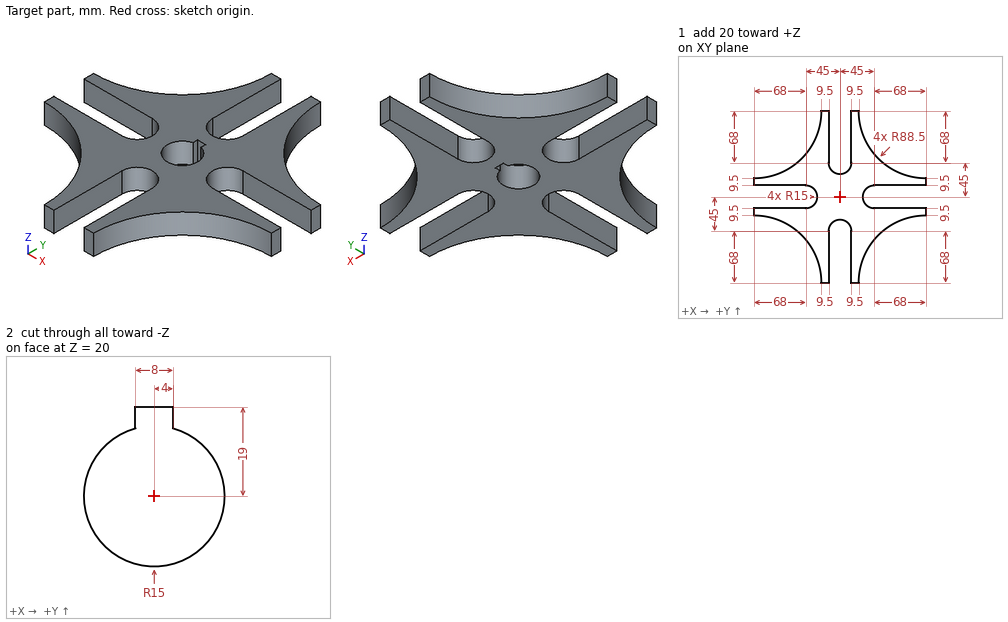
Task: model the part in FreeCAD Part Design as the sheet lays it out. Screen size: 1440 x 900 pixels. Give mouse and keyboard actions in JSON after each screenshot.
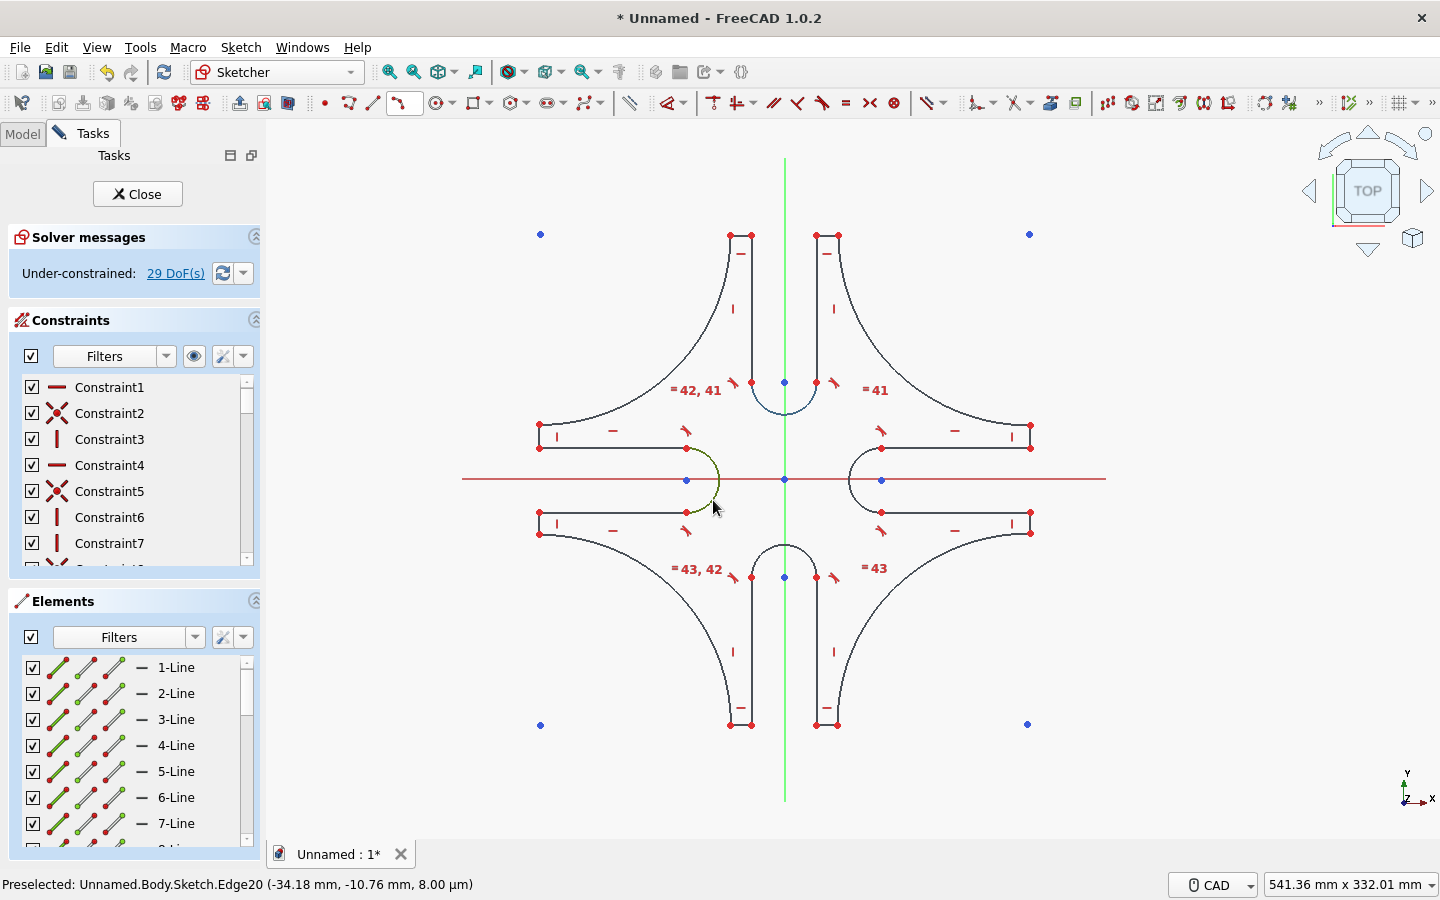
{"action": "left_click", "coordinate": [803, 551]}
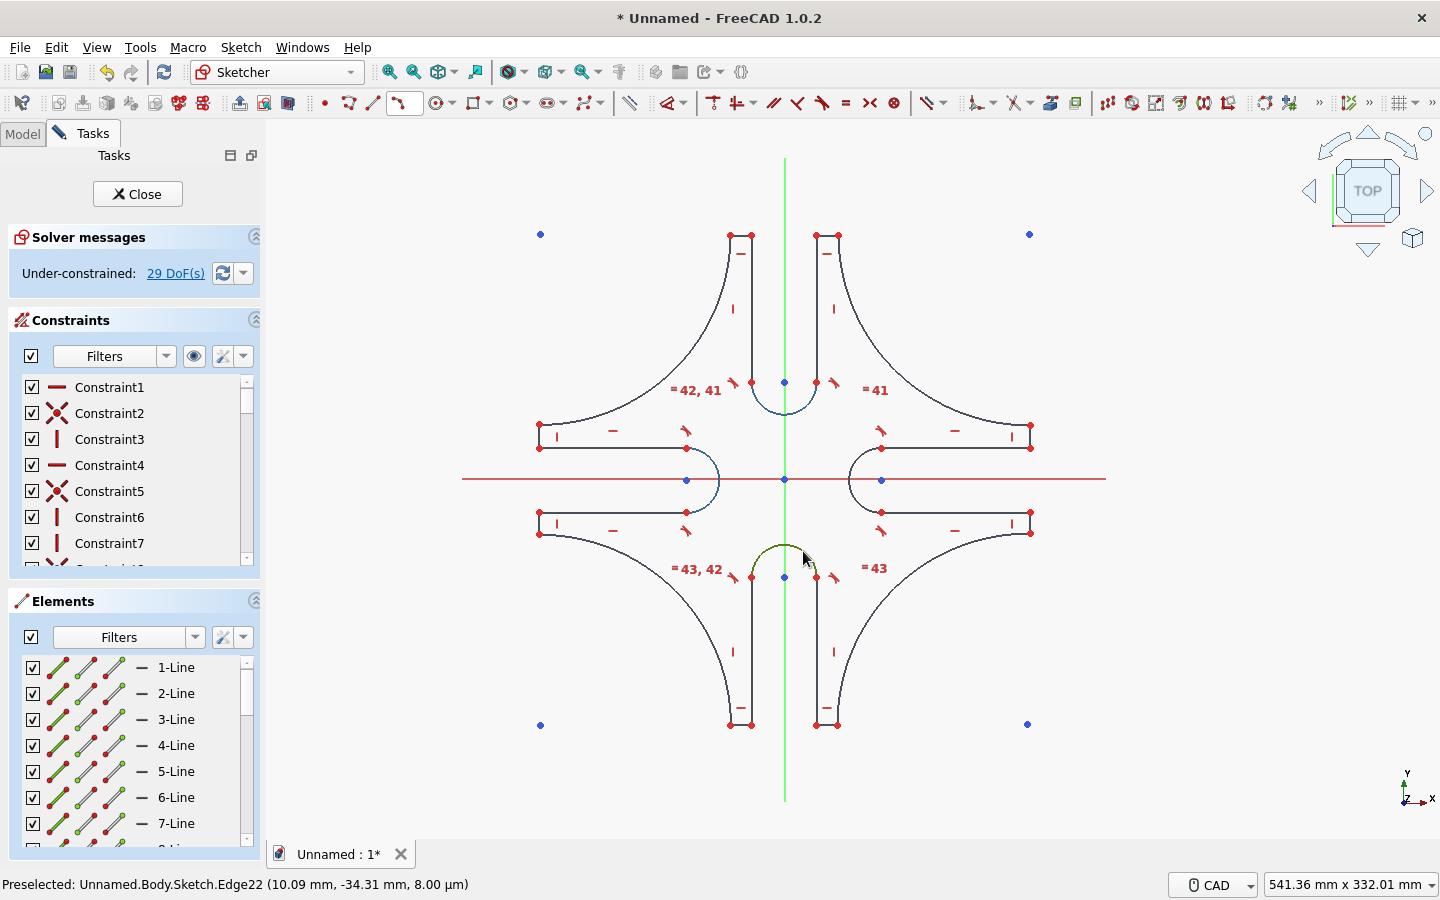
{"action": "left_click", "coordinate": [855, 461]}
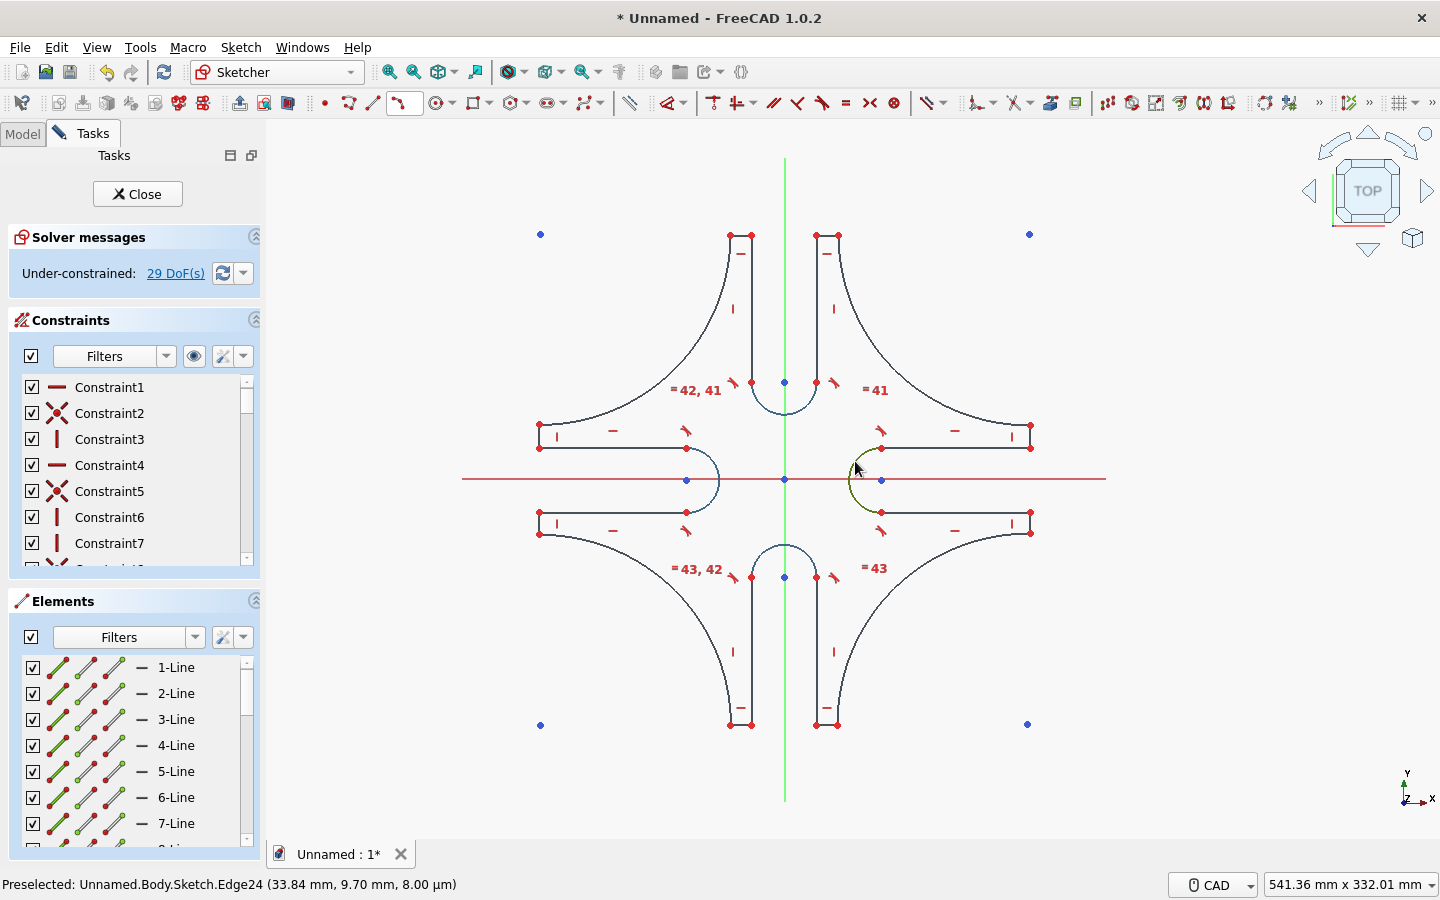
{"action": "left_click", "coordinate": [846, 104]}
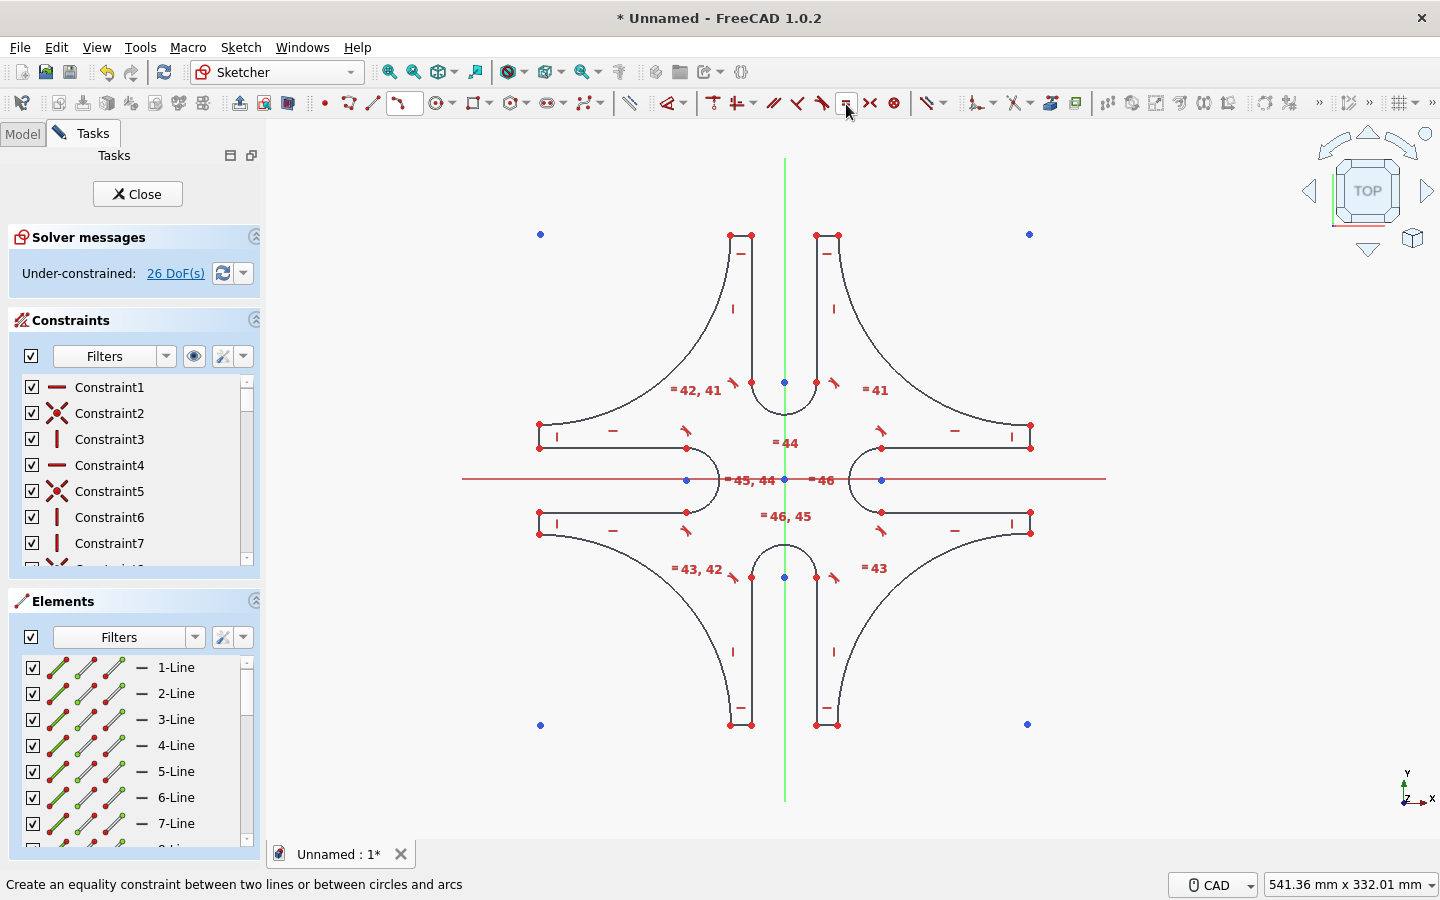
{"action": "left_click", "coordinate": [784, 382]}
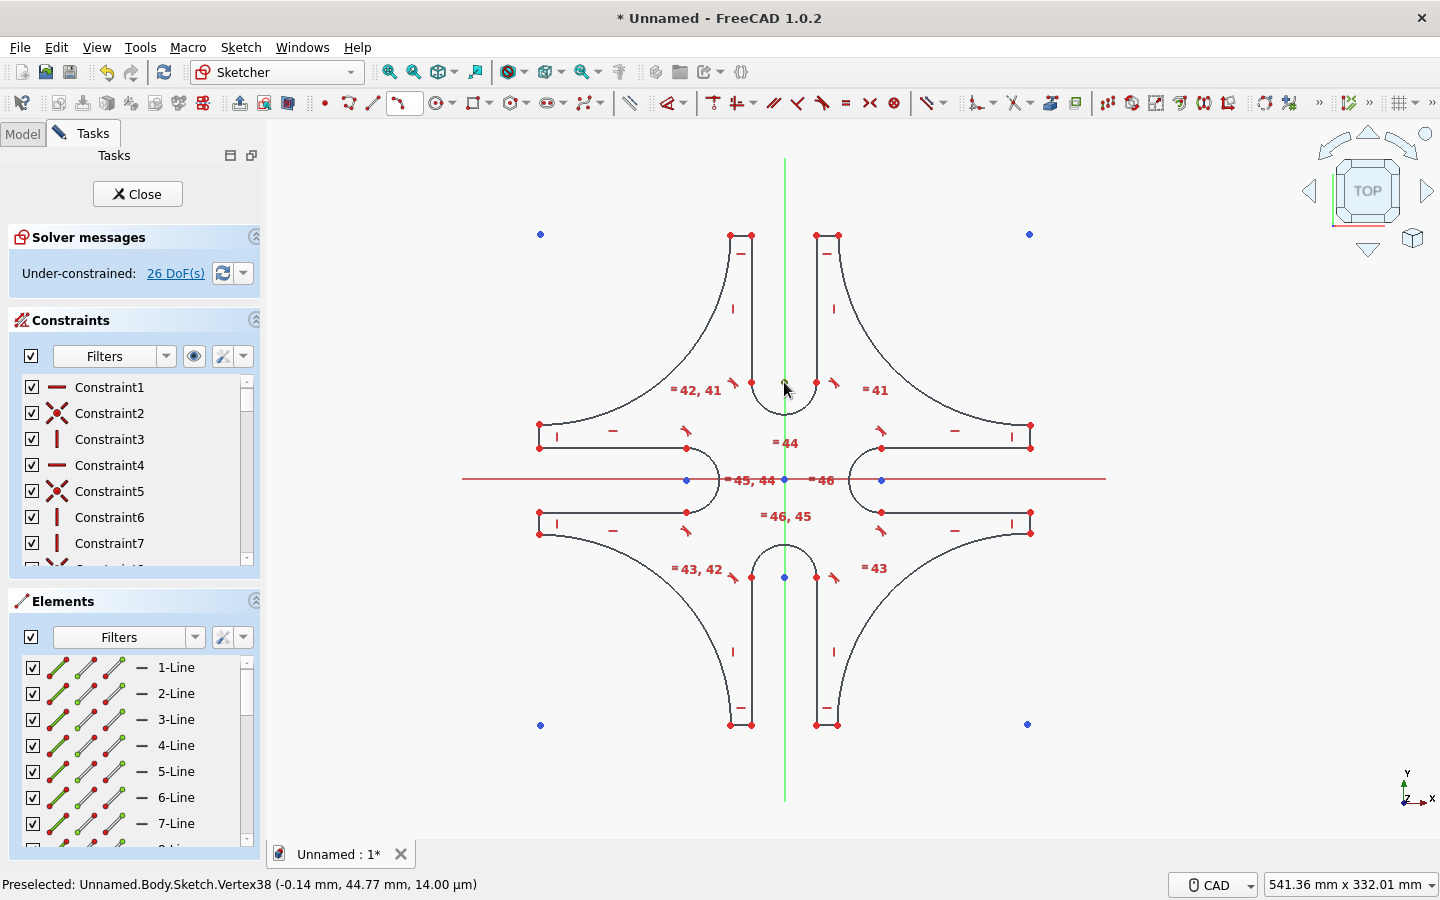
{"action": "left_click", "coordinate": [785, 764]}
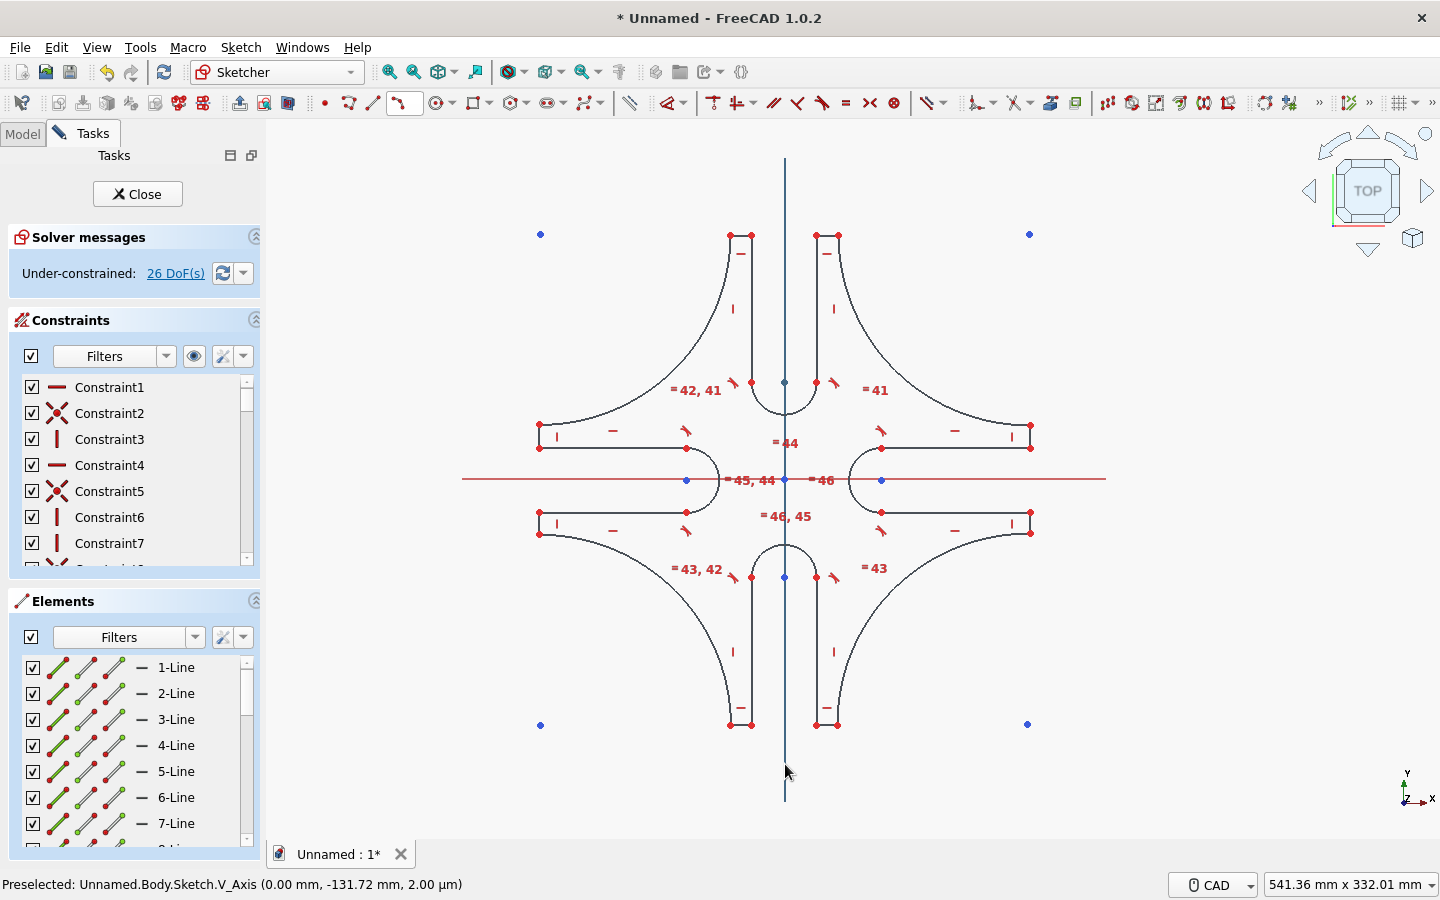
{"action": "left_click", "coordinate": [714, 104]}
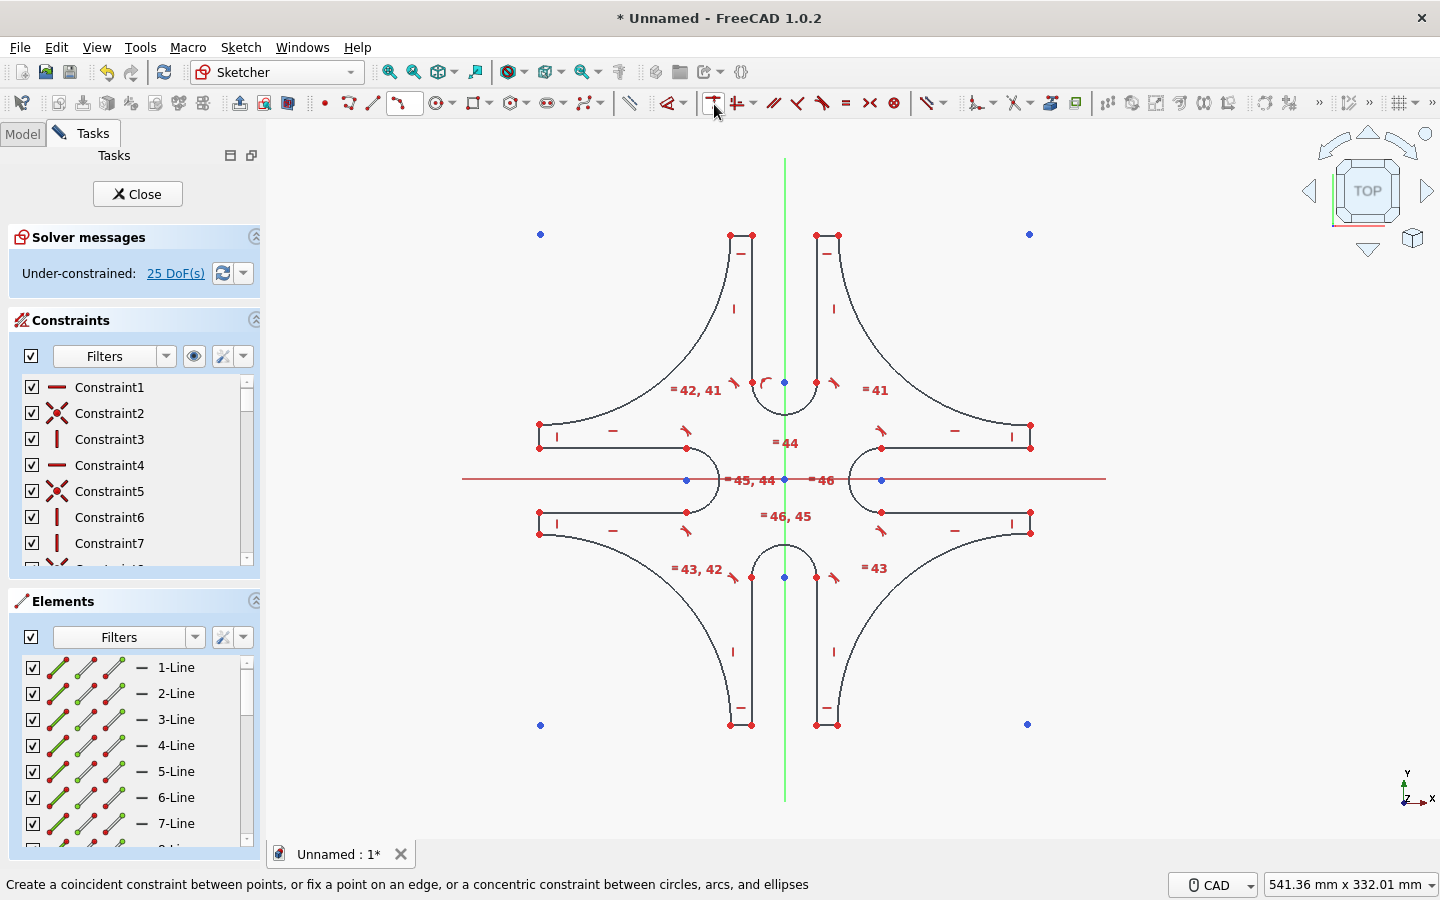
{"action": "left_click", "coordinate": [687, 480]}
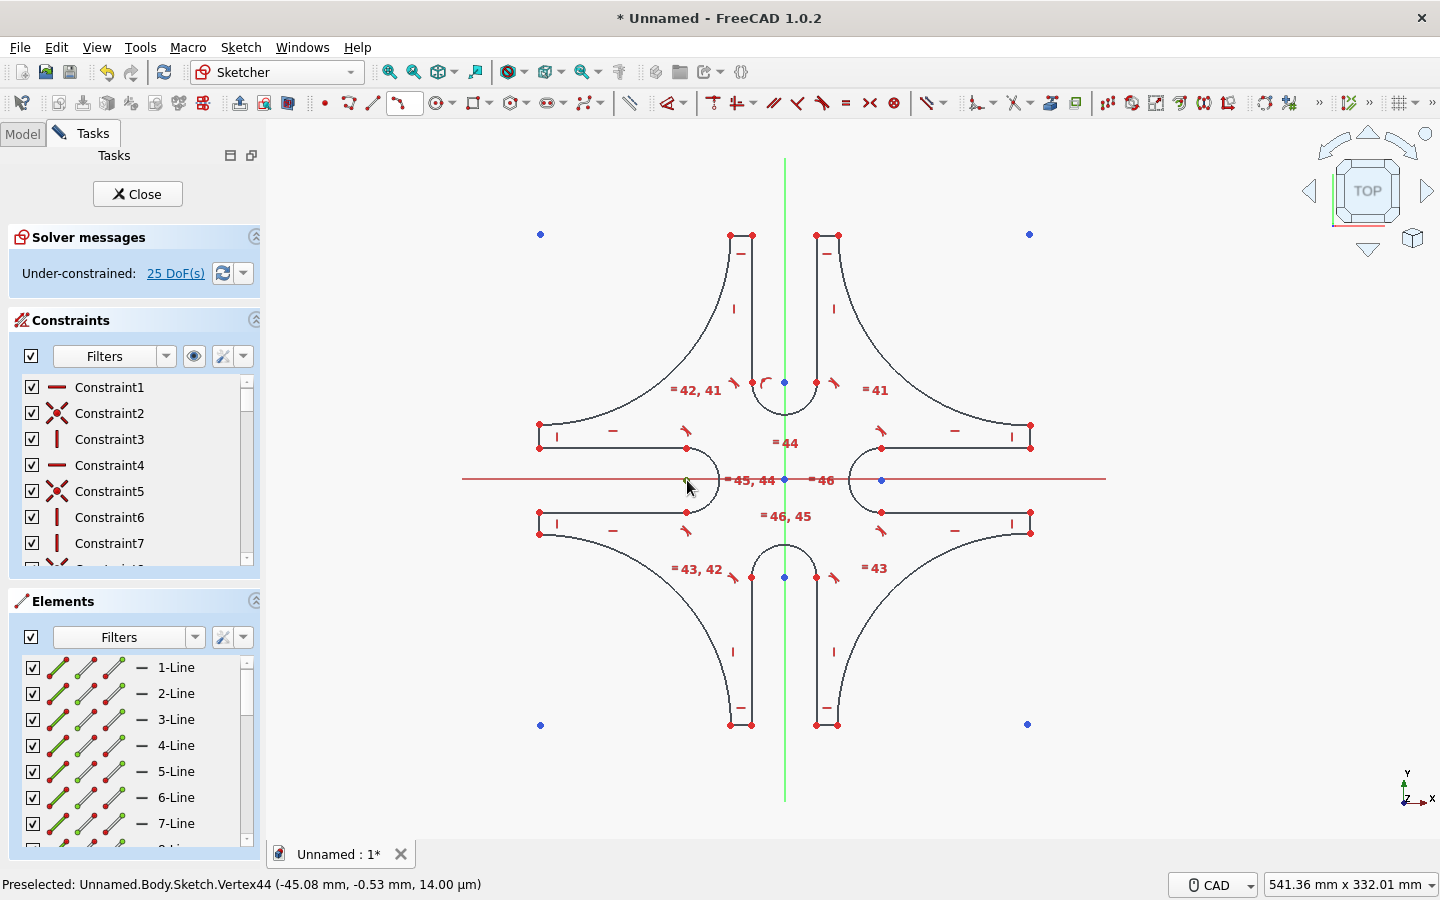
{"action": "left_click", "coordinate": [504, 479]}